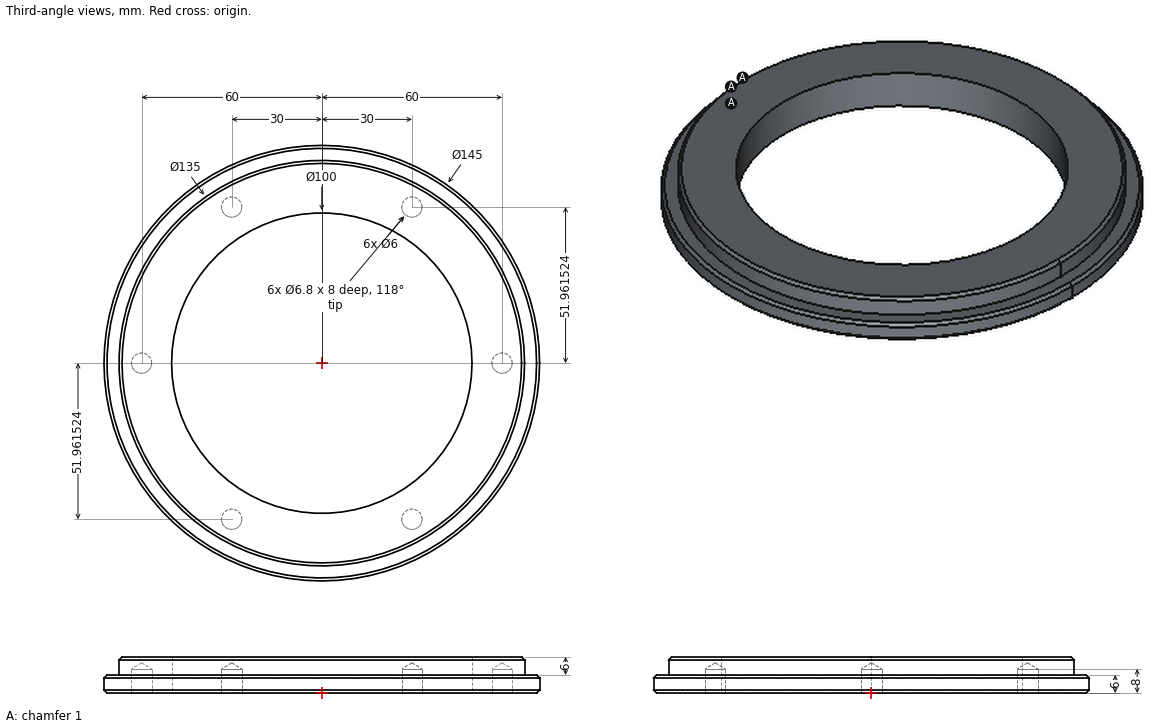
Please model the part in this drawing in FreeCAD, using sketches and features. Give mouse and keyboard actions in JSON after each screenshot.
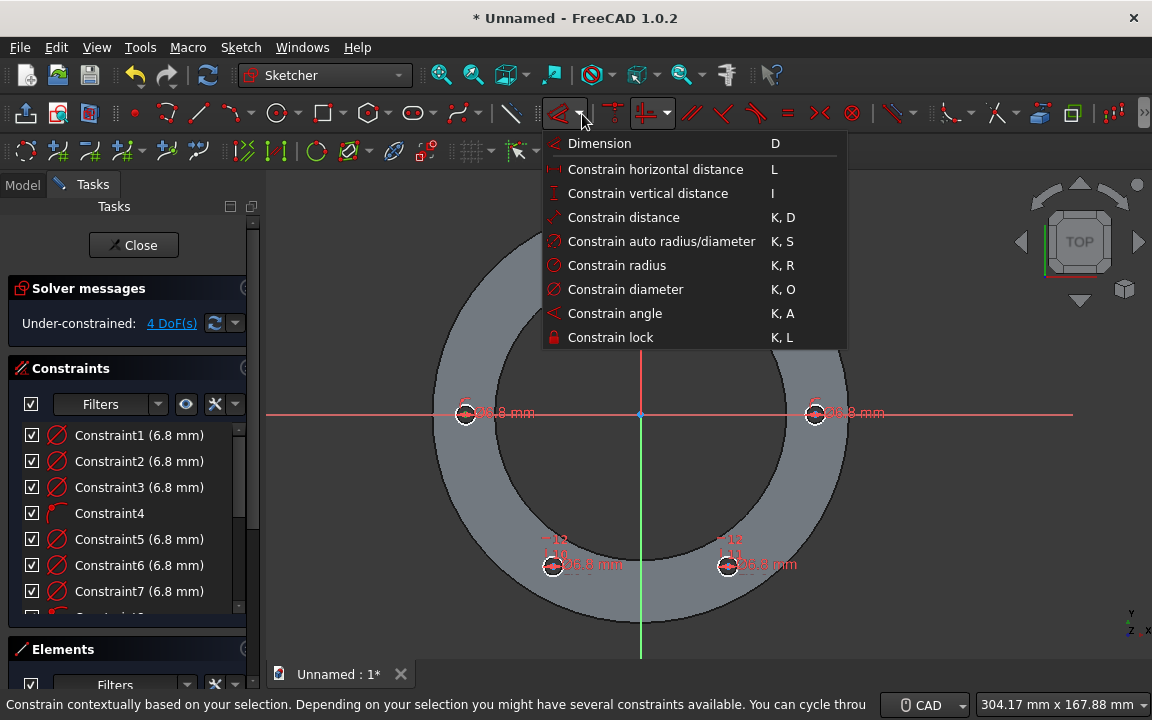
{"action": "left_click", "coordinate": [695, 169]}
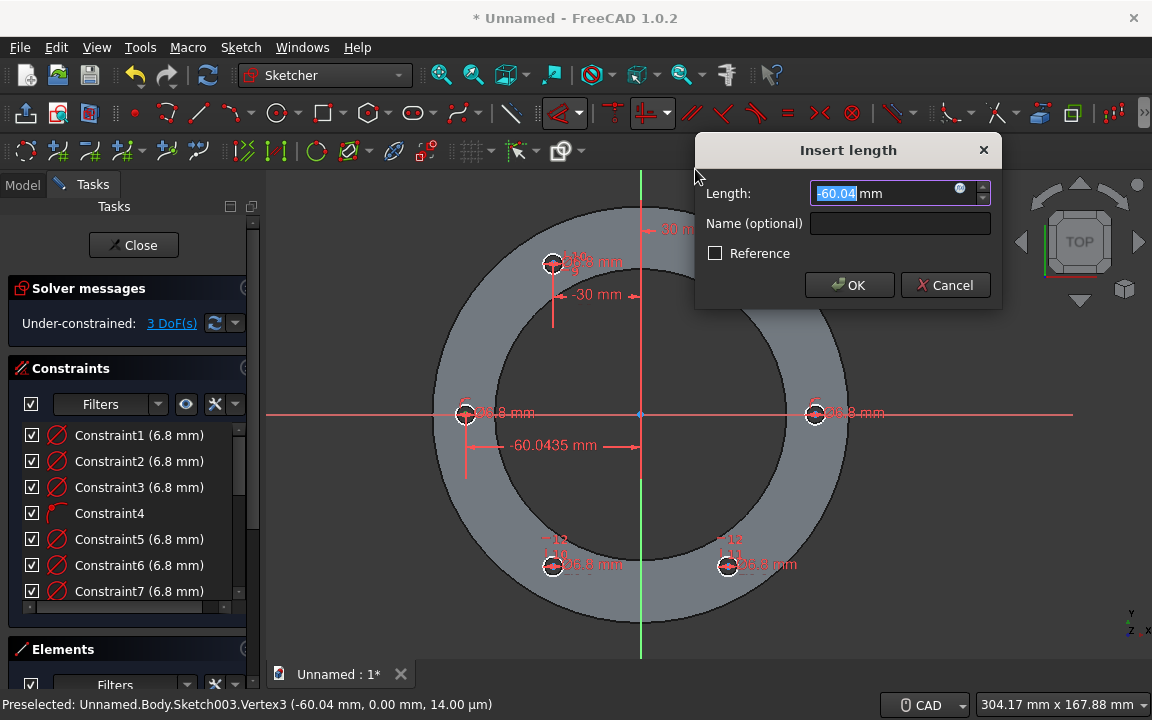
{"action": "type", "text": "-60"}
{"action": "key", "text": "Return"}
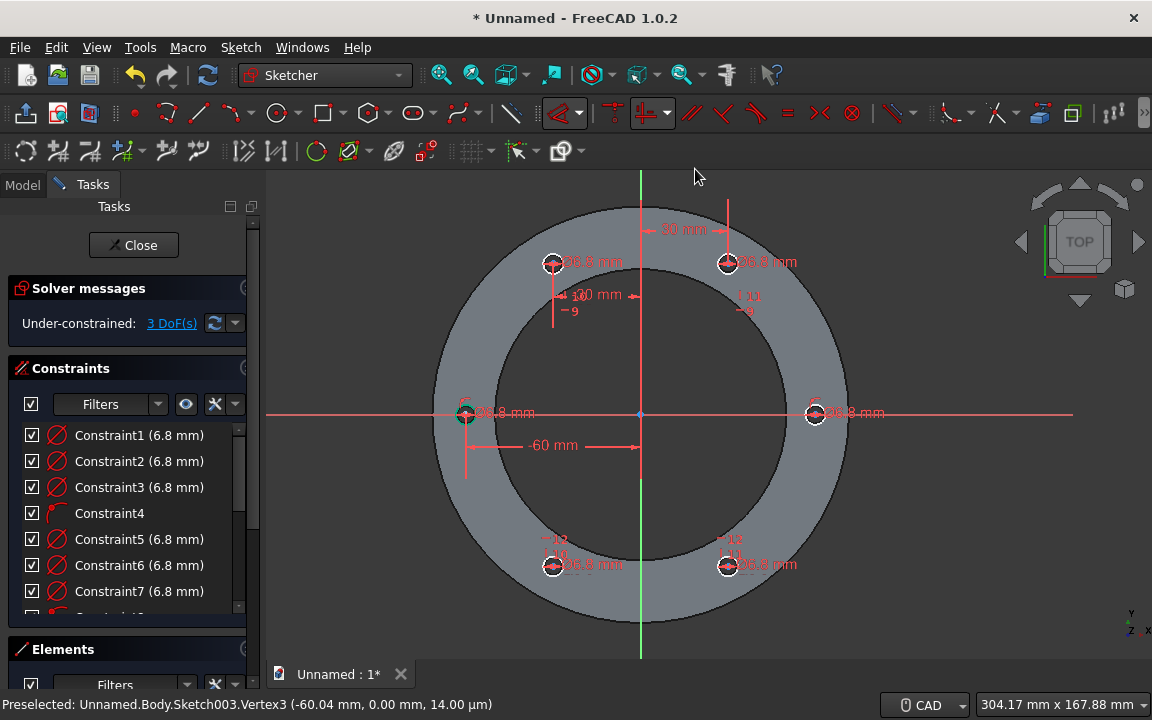
{"action": "left_click", "coordinate": [815, 415]}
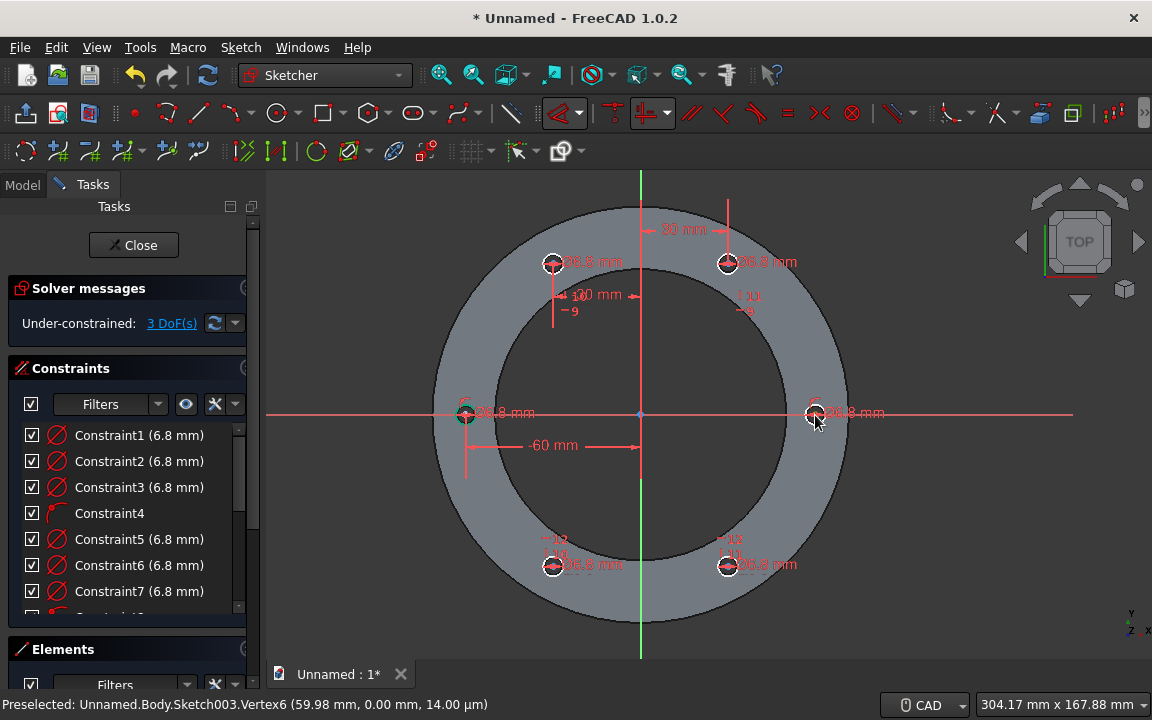
{"action": "key", "text": "l"}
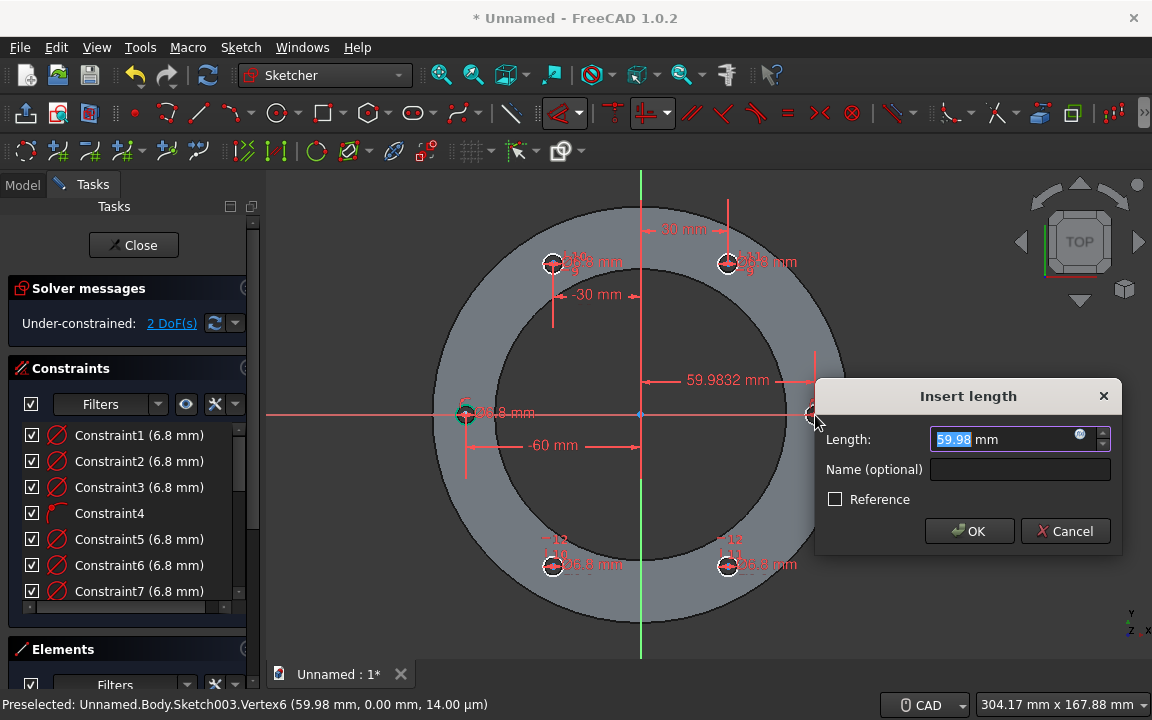
{"action": "type", "text": "60"}
{"action": "key", "text": "Return"}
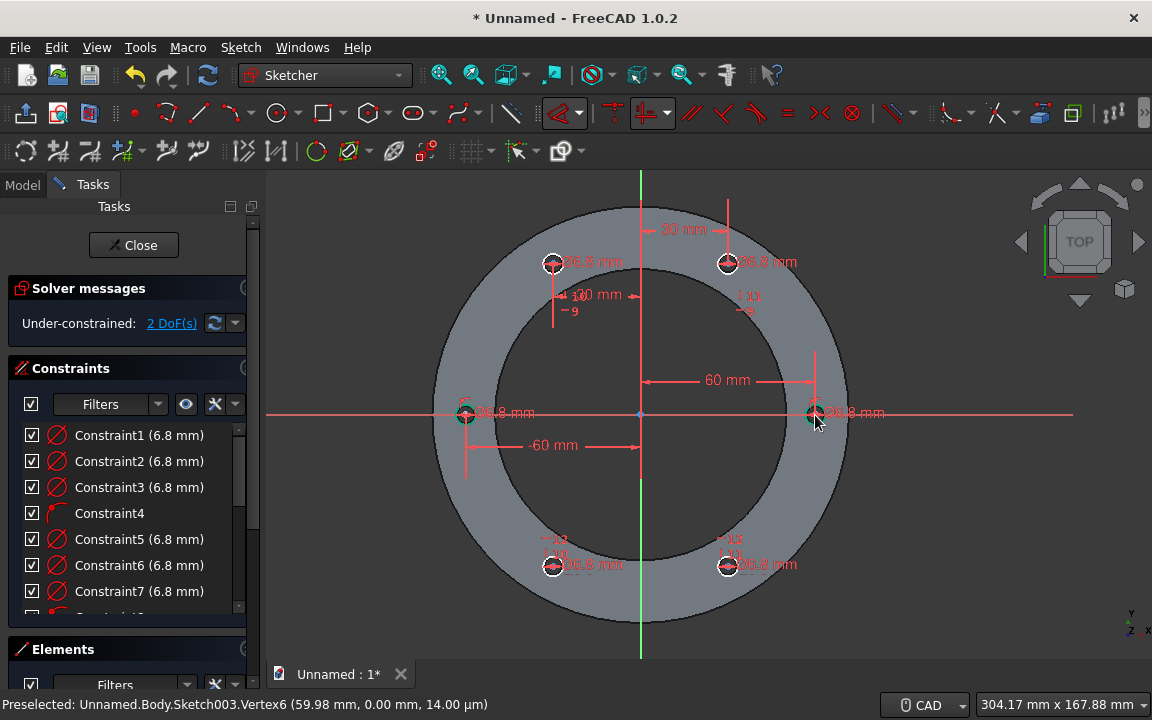
{"action": "left_click", "coordinate": [728, 264]}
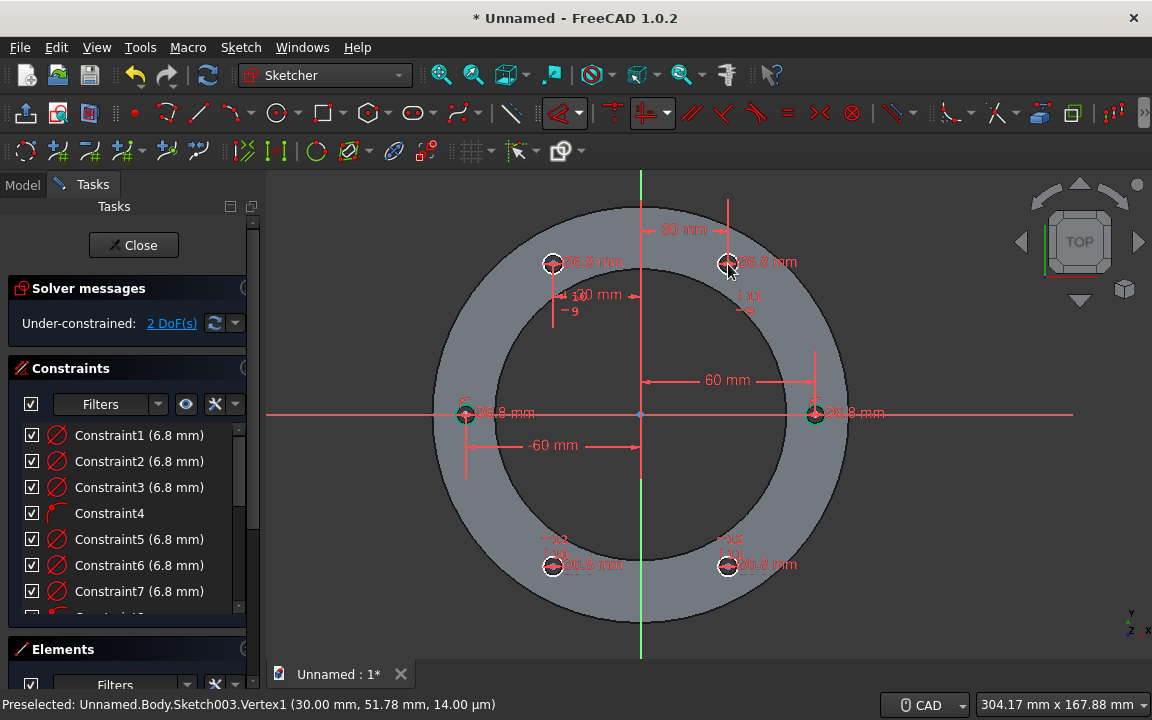
{"action": "key", "text": "i"}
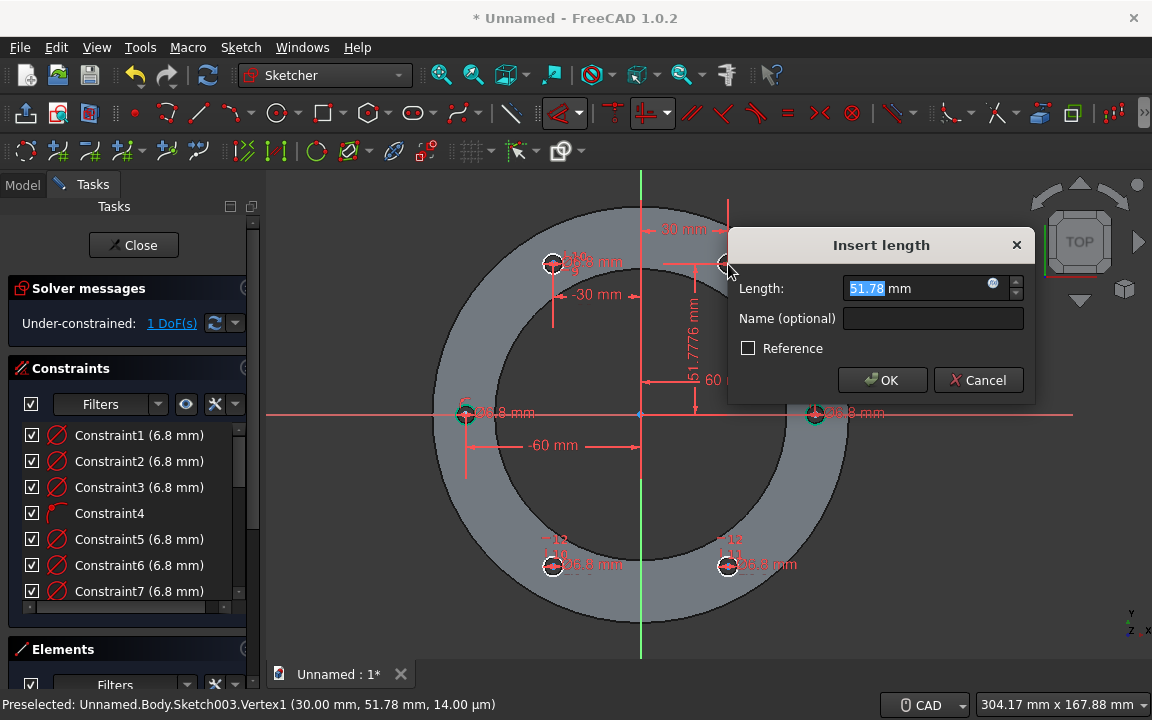
{"action": "type", "text": "51.961524"}
{"action": "key", "text": "Return"}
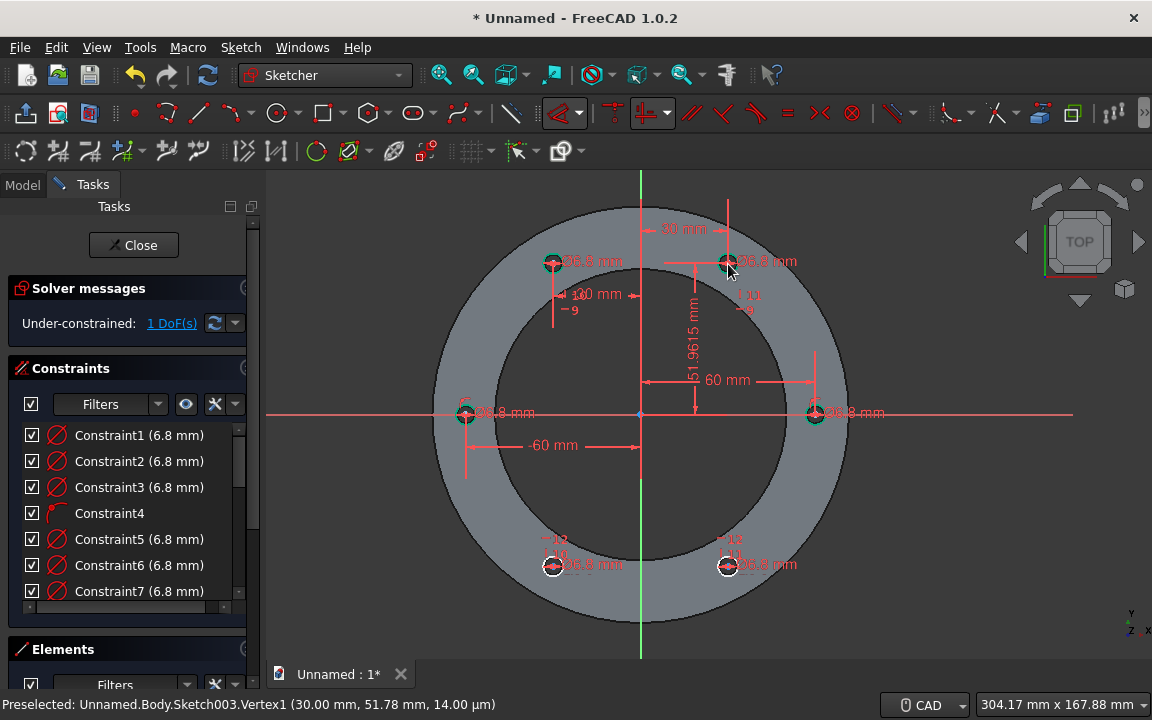
{"action": "left_click", "coordinate": [553, 567]}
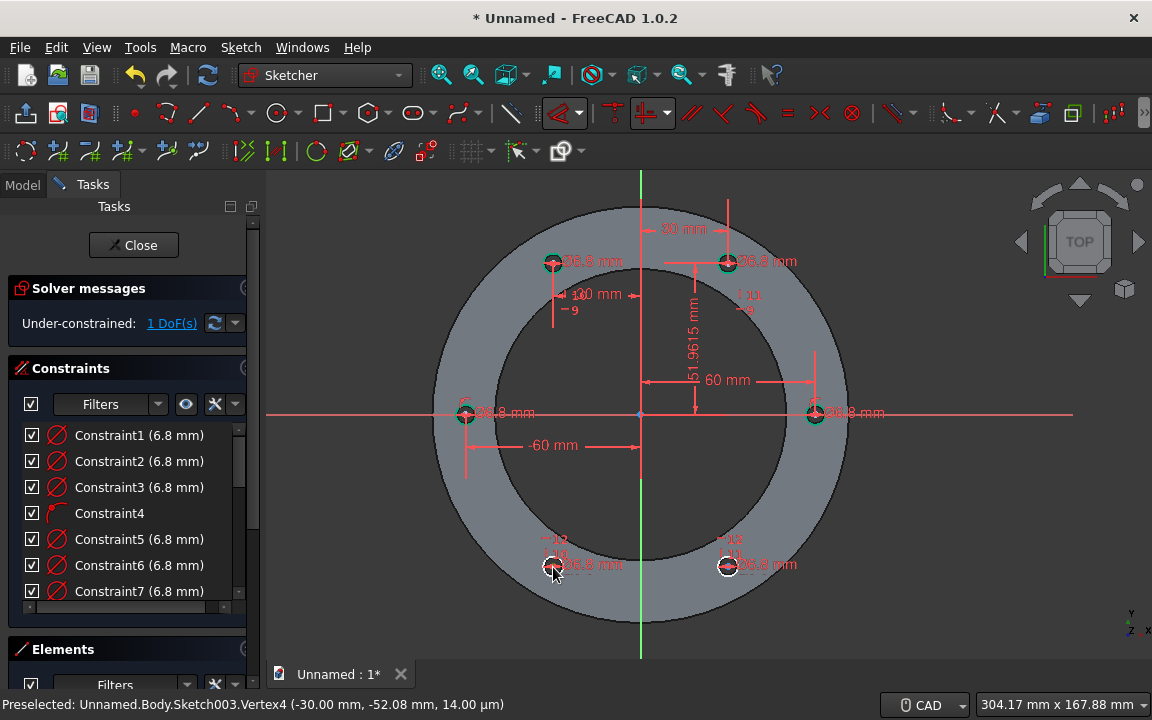
{"action": "left_click", "coordinate": [582, 114]}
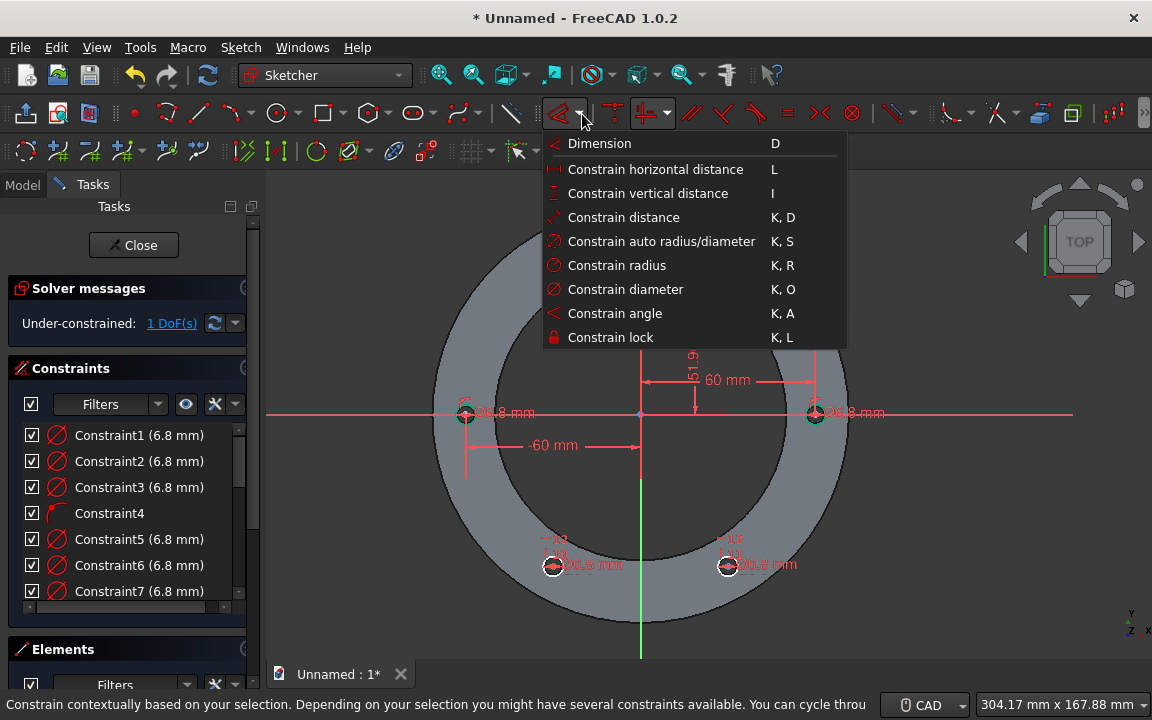
{"action": "left_click", "coordinate": [695, 193]}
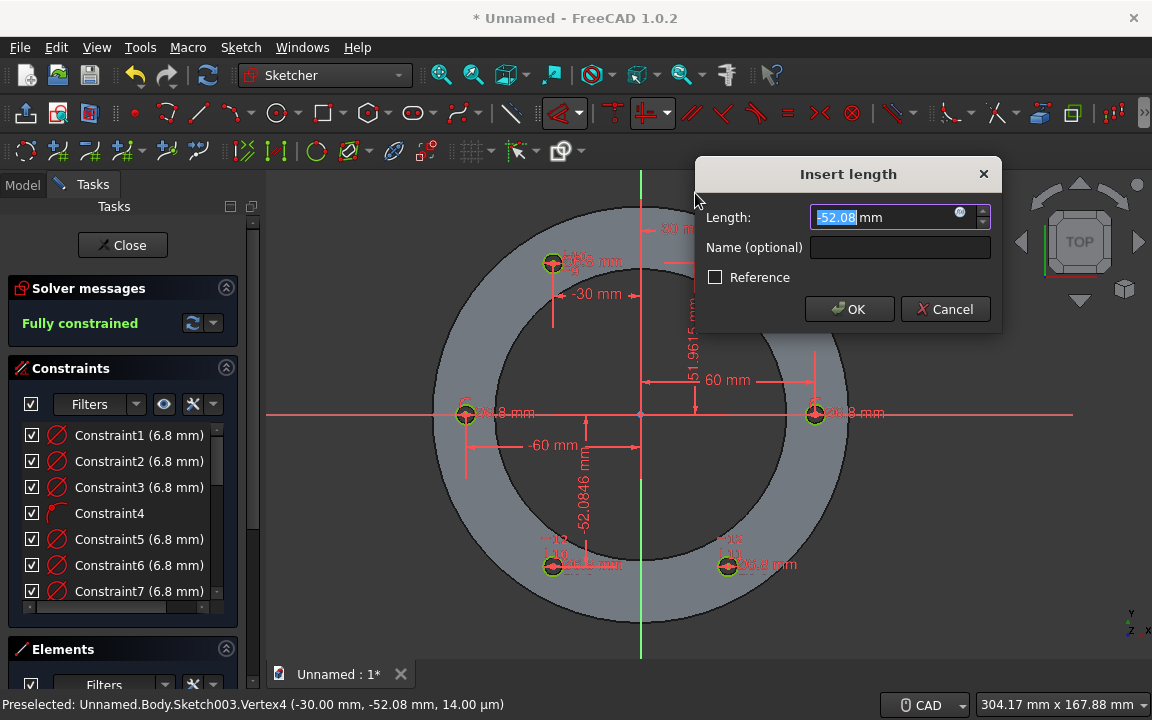
{"action": "type", "text": "-51.961524"}
{"action": "key", "text": "Return"}